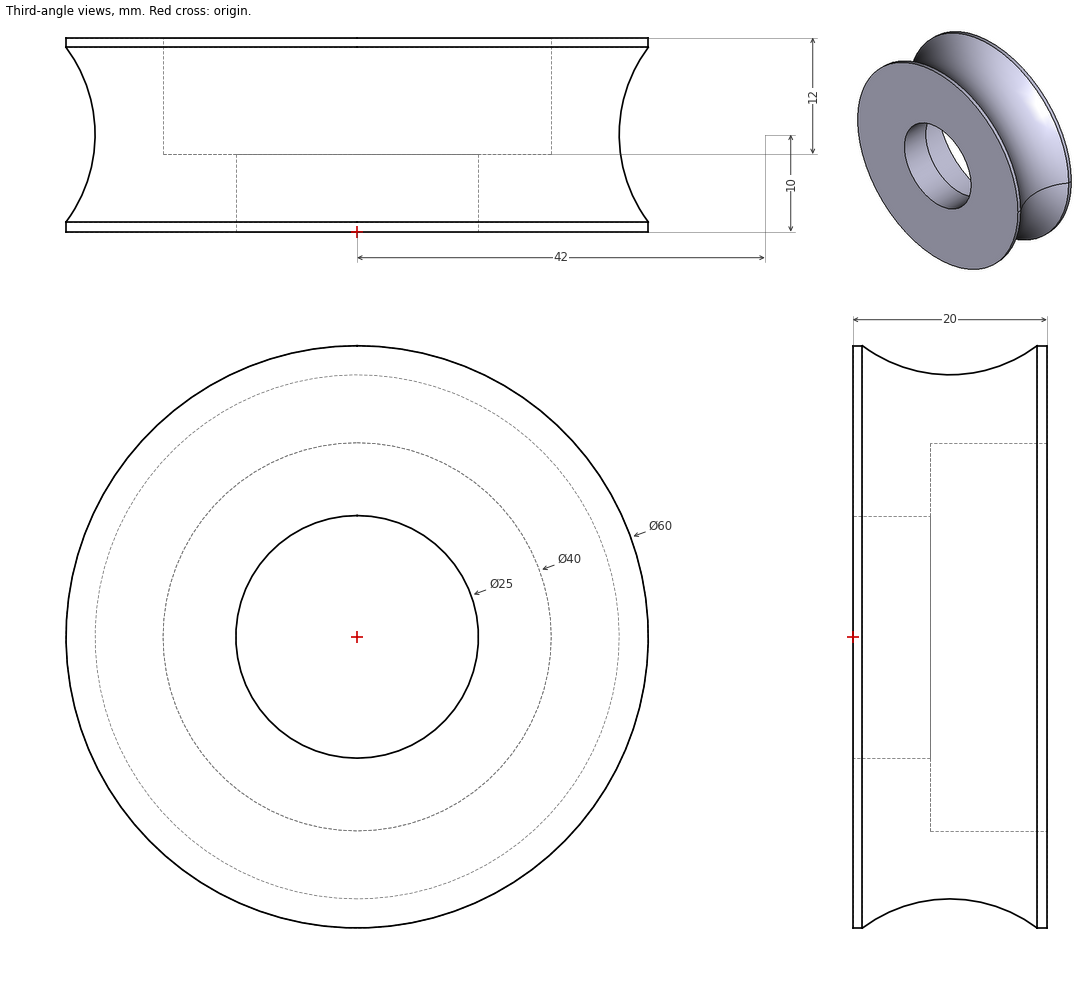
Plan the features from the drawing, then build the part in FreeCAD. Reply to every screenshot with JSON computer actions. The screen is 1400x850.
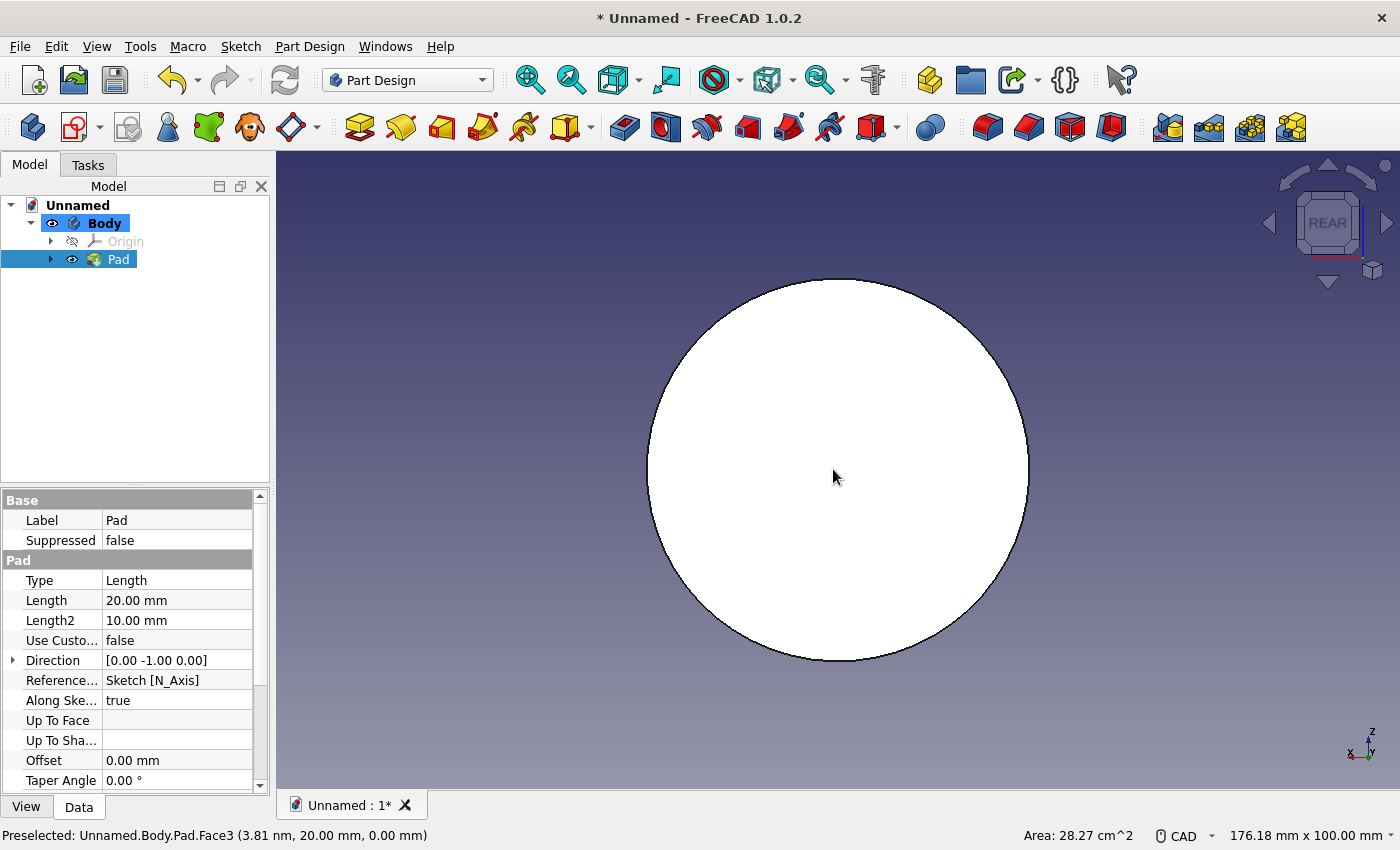
{"action": "left_click", "coordinate": [74, 128]}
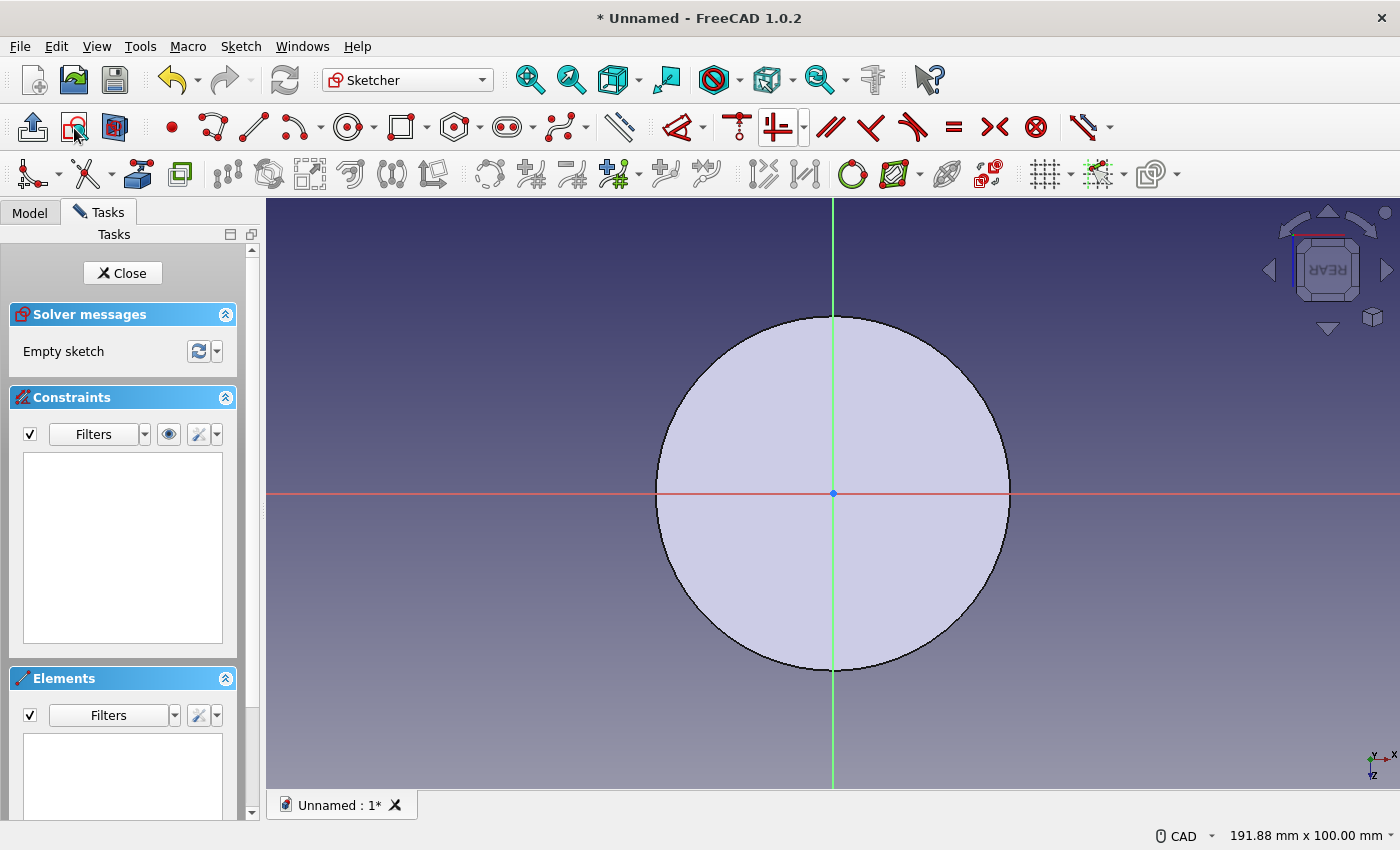
{"action": "scroll", "coordinate": [972, 494], "scroll_direction": "up", "scroll_amount": 2}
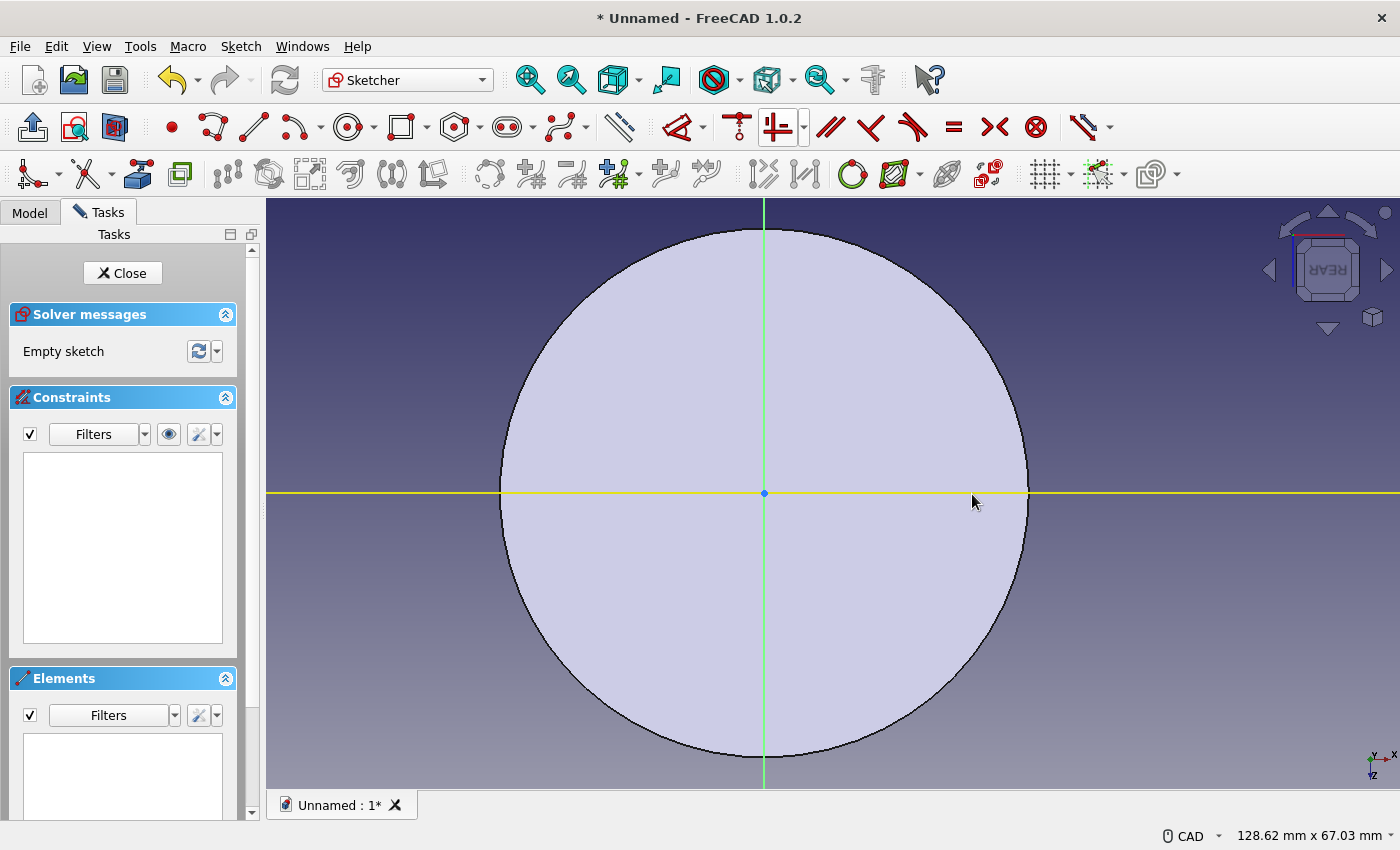
{"action": "left_click", "coordinate": [348, 128]}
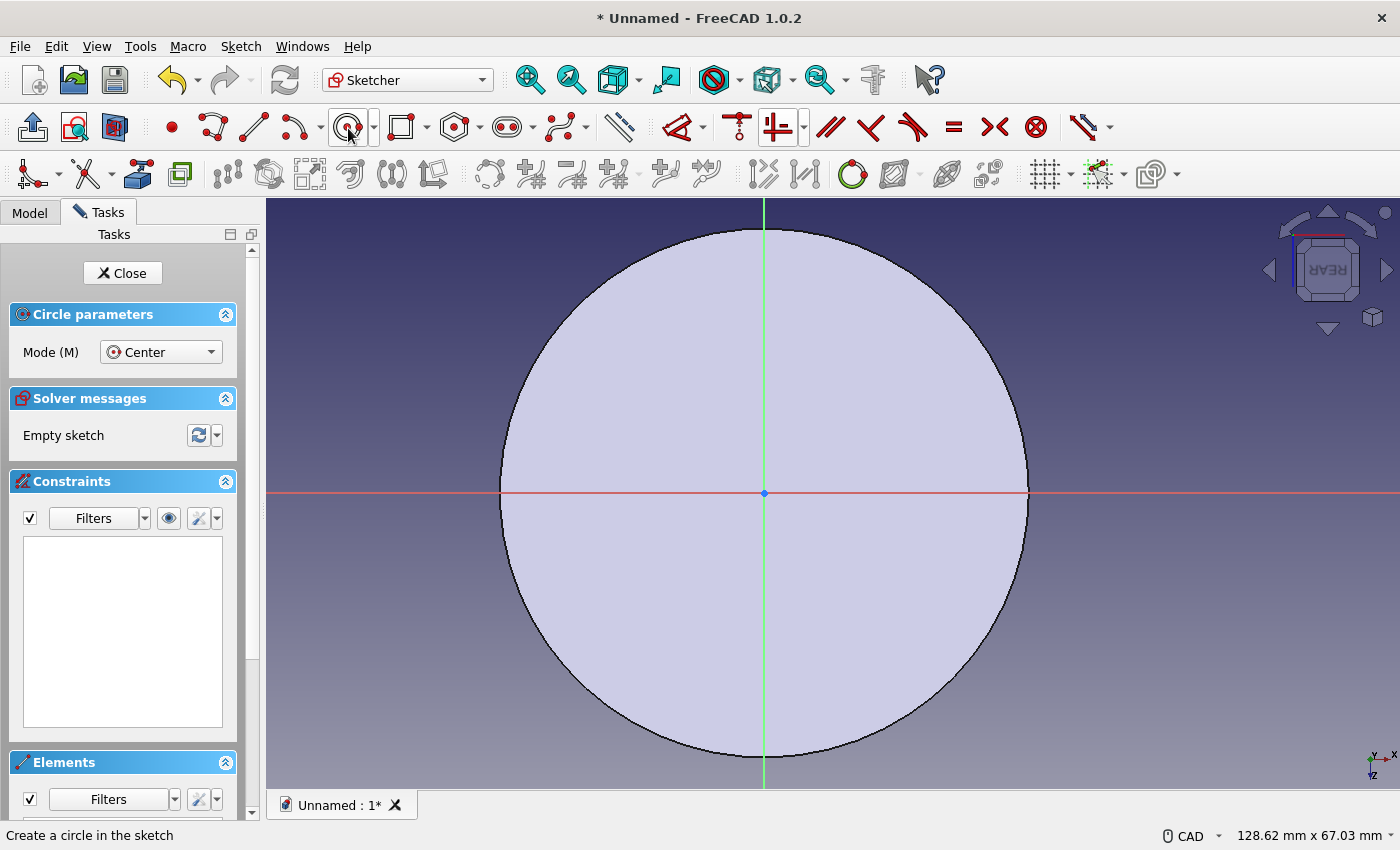
{"action": "left_click", "coordinate": [764, 493]}
{"action": "left_click", "coordinate": [889, 368]}
{"action": "key", "text": "Escape"}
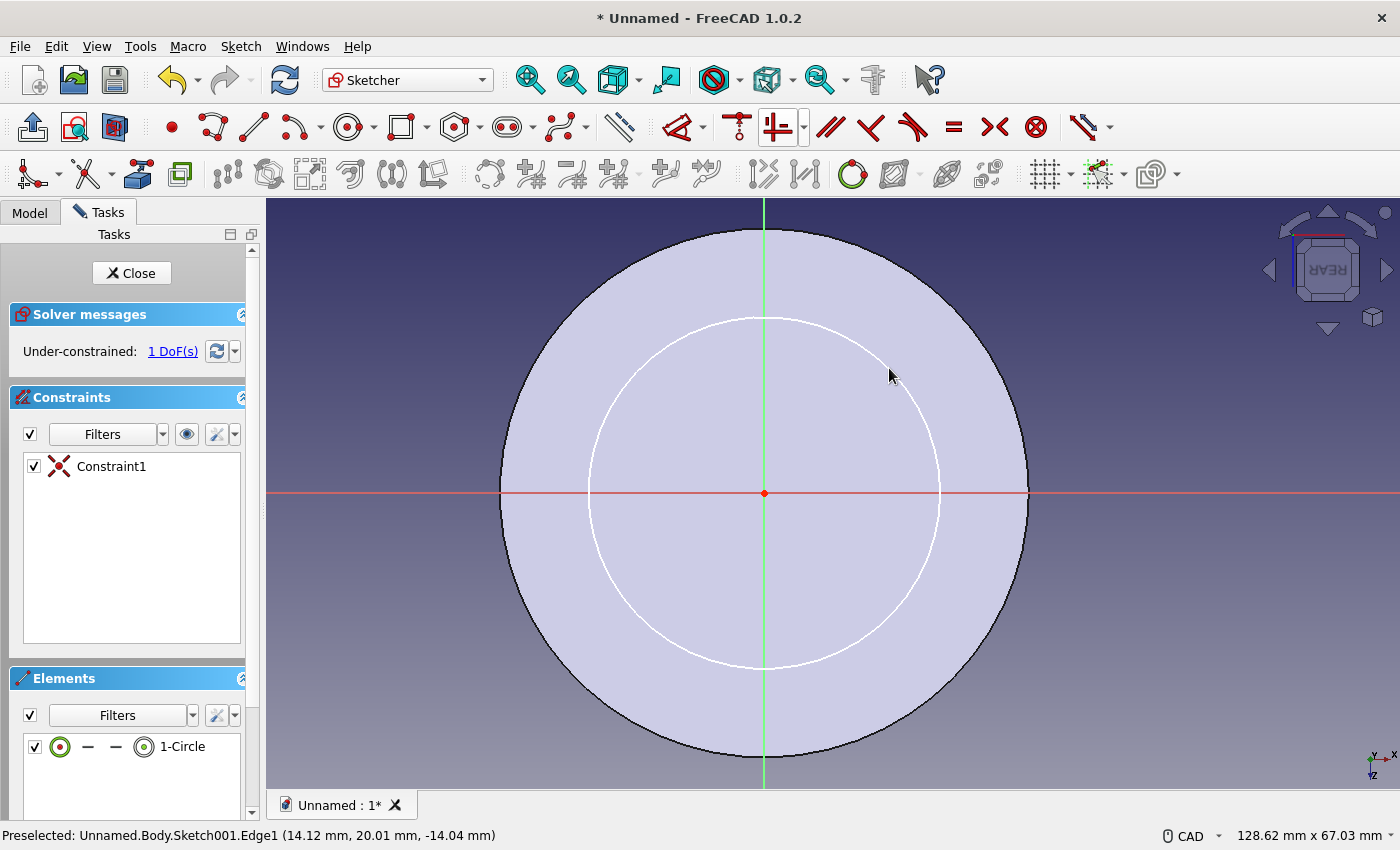
{"action": "left_click", "coordinate": [676, 128]}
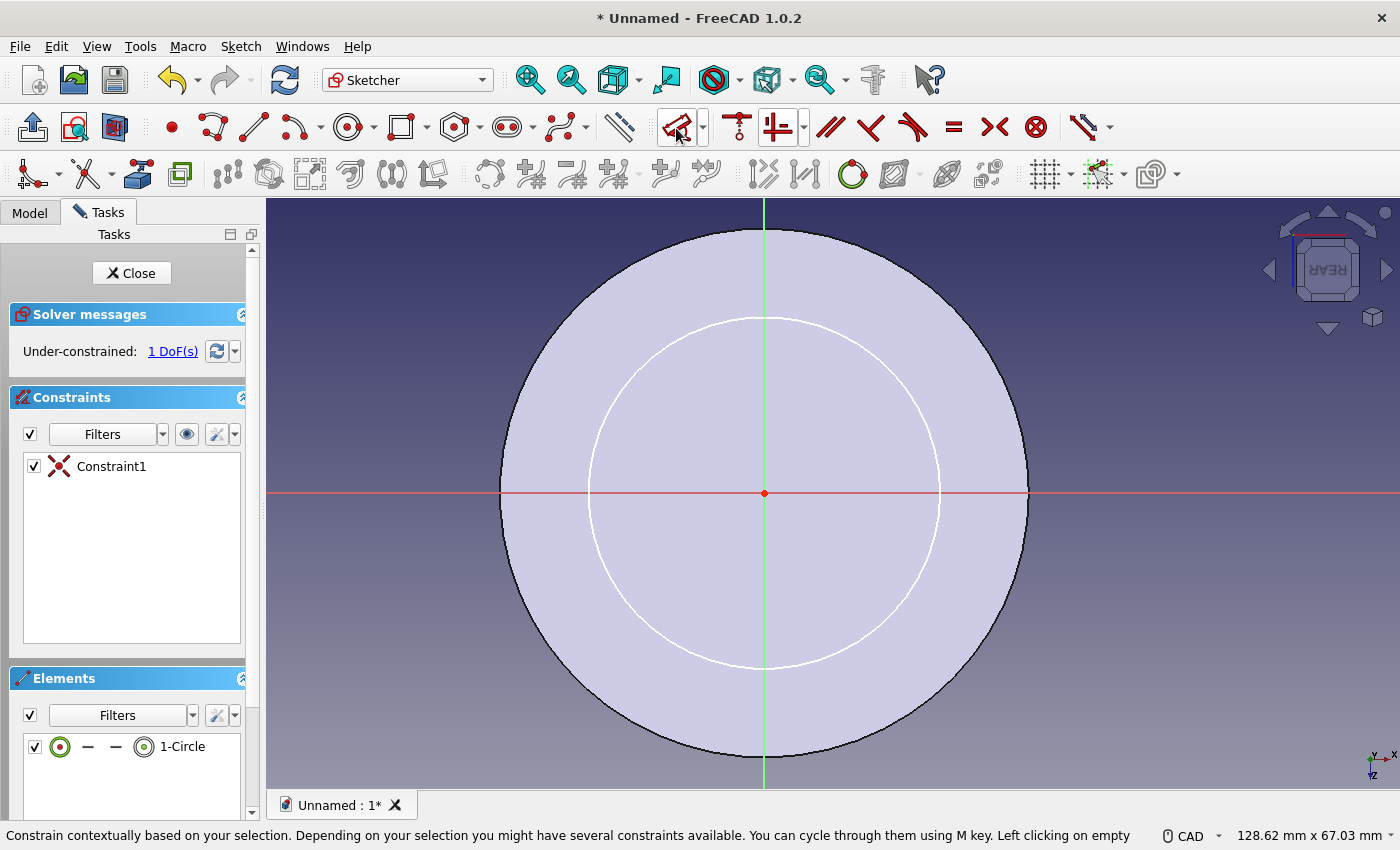
{"action": "left_click", "coordinate": [888, 368]}
{"action": "left_click", "coordinate": [911, 345]}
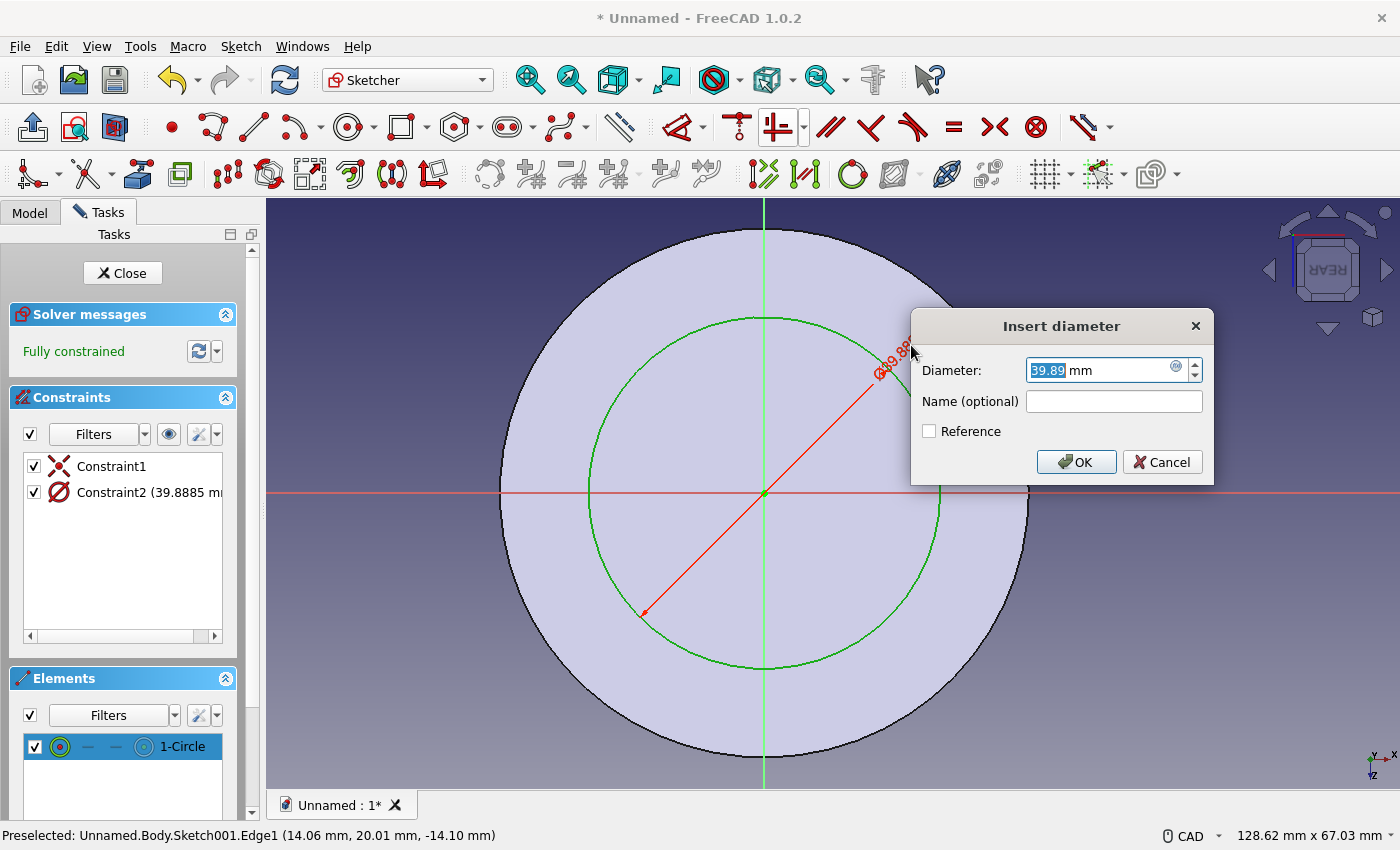
{"action": "type", "text": "40"}
{"action": "key", "text": "Return"}
{"action": "key", "text": "Escape"}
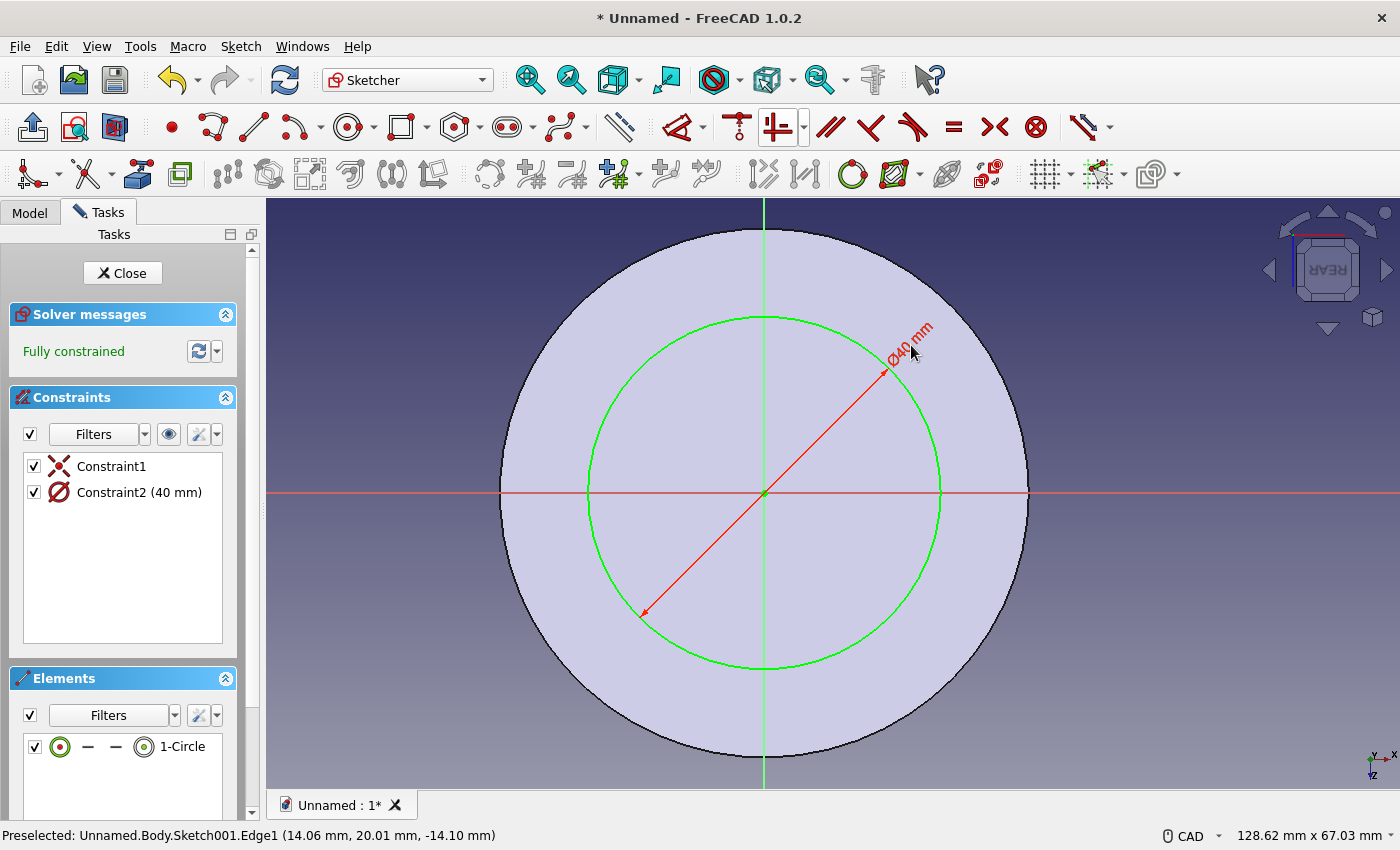
{"action": "left_click", "coordinate": [123, 273]}